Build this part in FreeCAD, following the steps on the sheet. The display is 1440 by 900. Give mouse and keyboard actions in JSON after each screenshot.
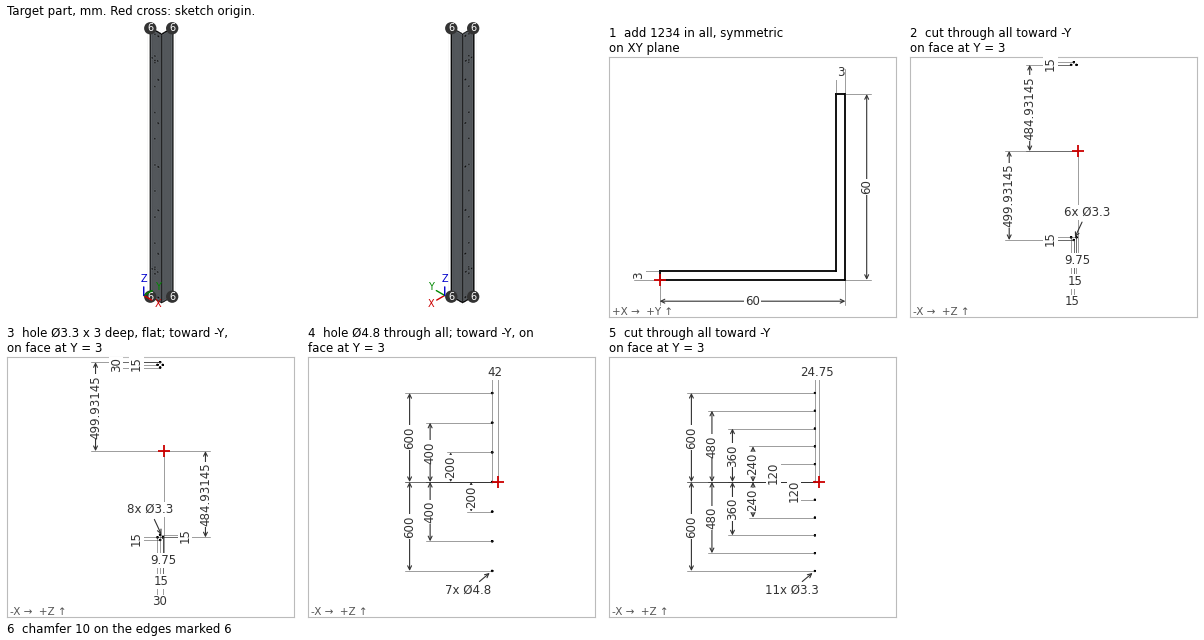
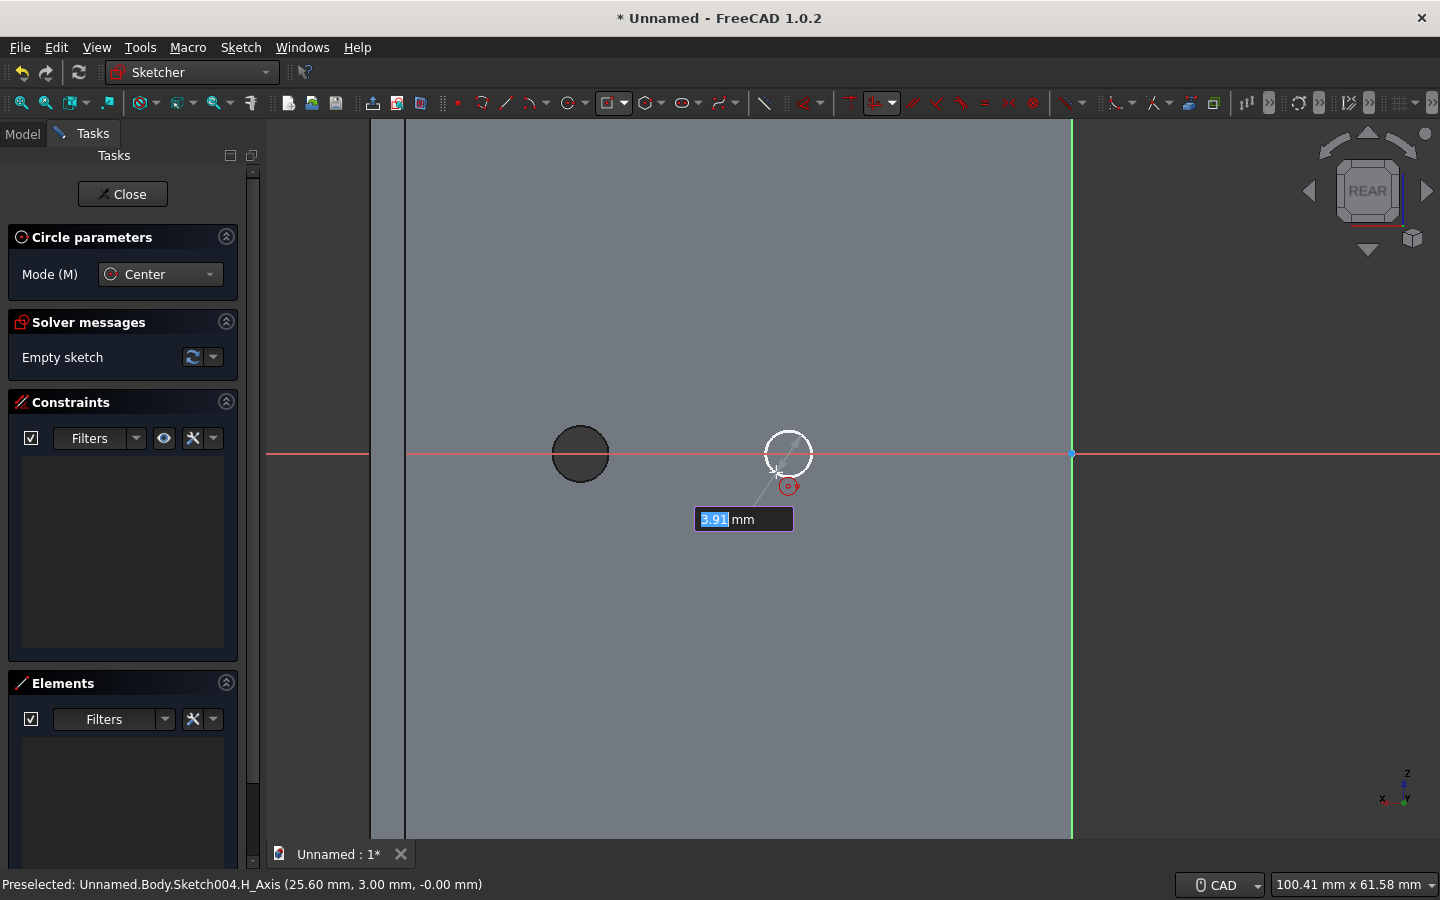
{"action": "type", "text": "3.3"}
{"action": "key", "text": "Return"}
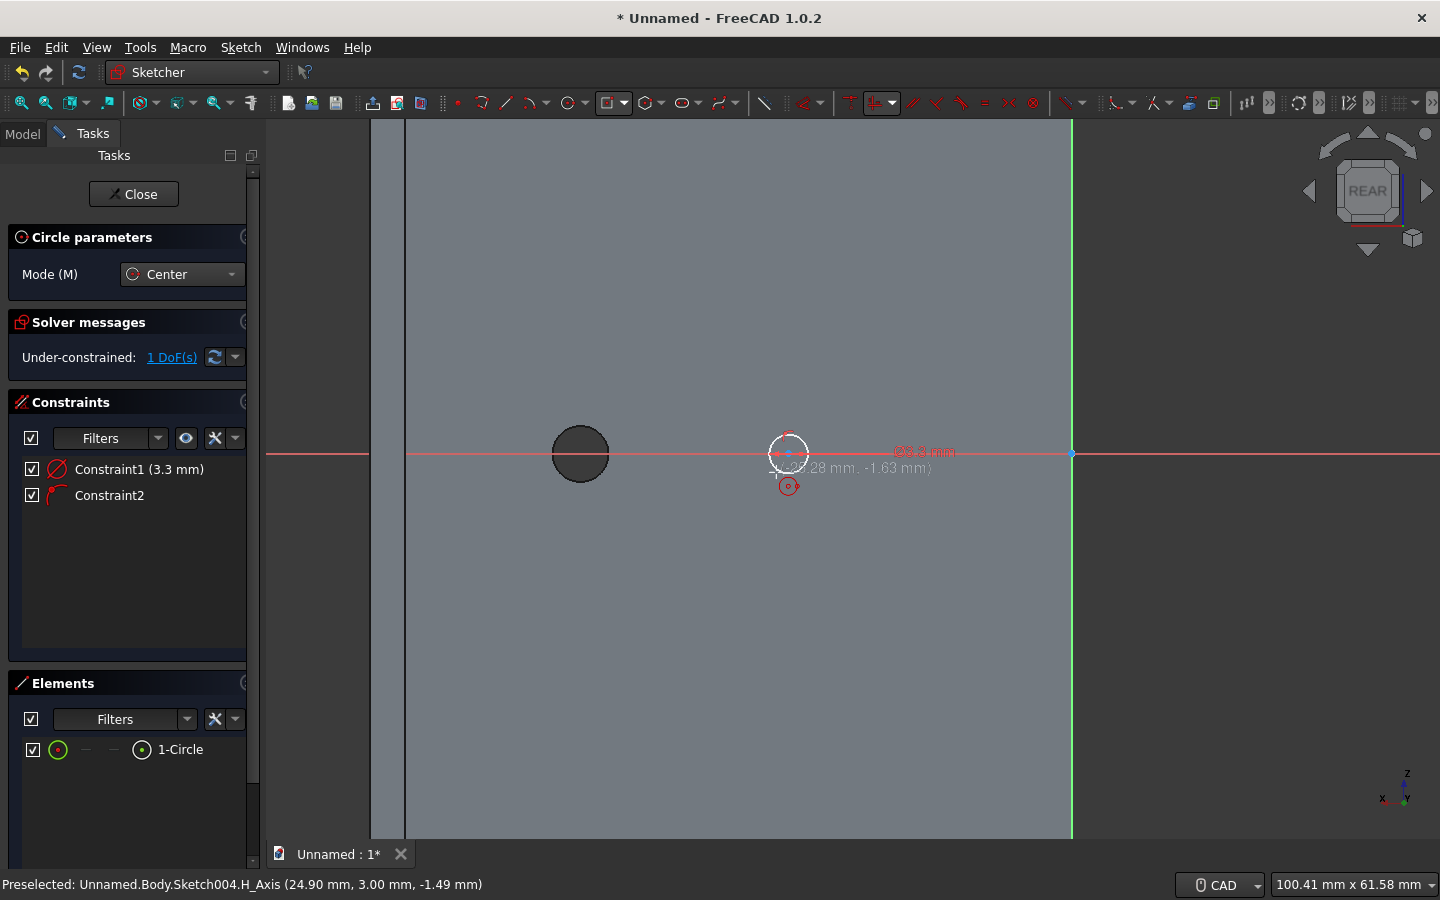
{"action": "scroll", "coordinate": [779, 480], "scroll_direction": "down", "scroll_amount": 16}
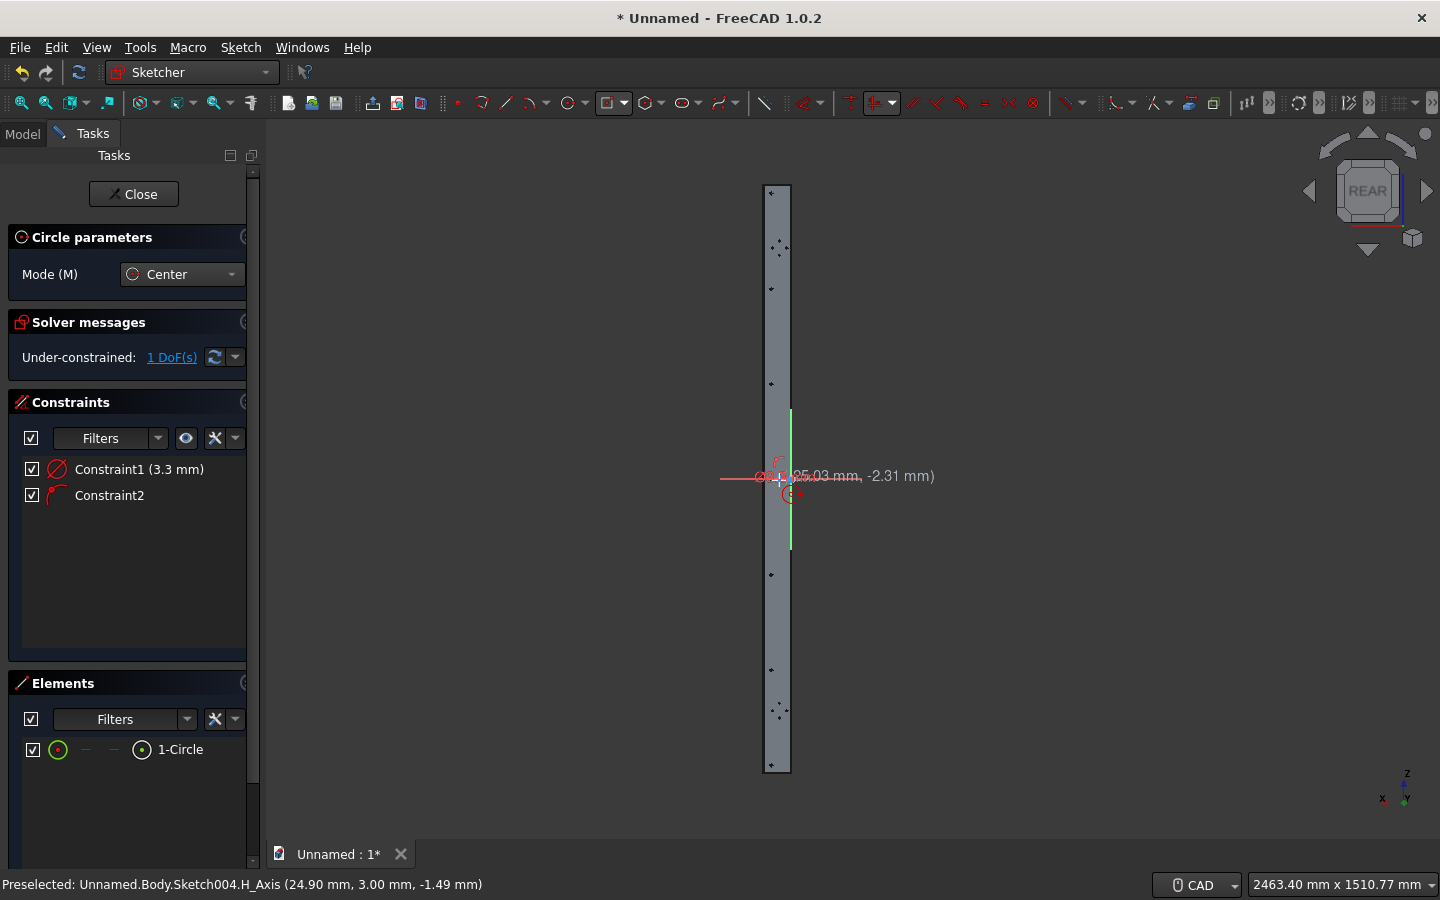
{"action": "scroll", "coordinate": [780, 537], "scroll_direction": "up", "scroll_amount": 17}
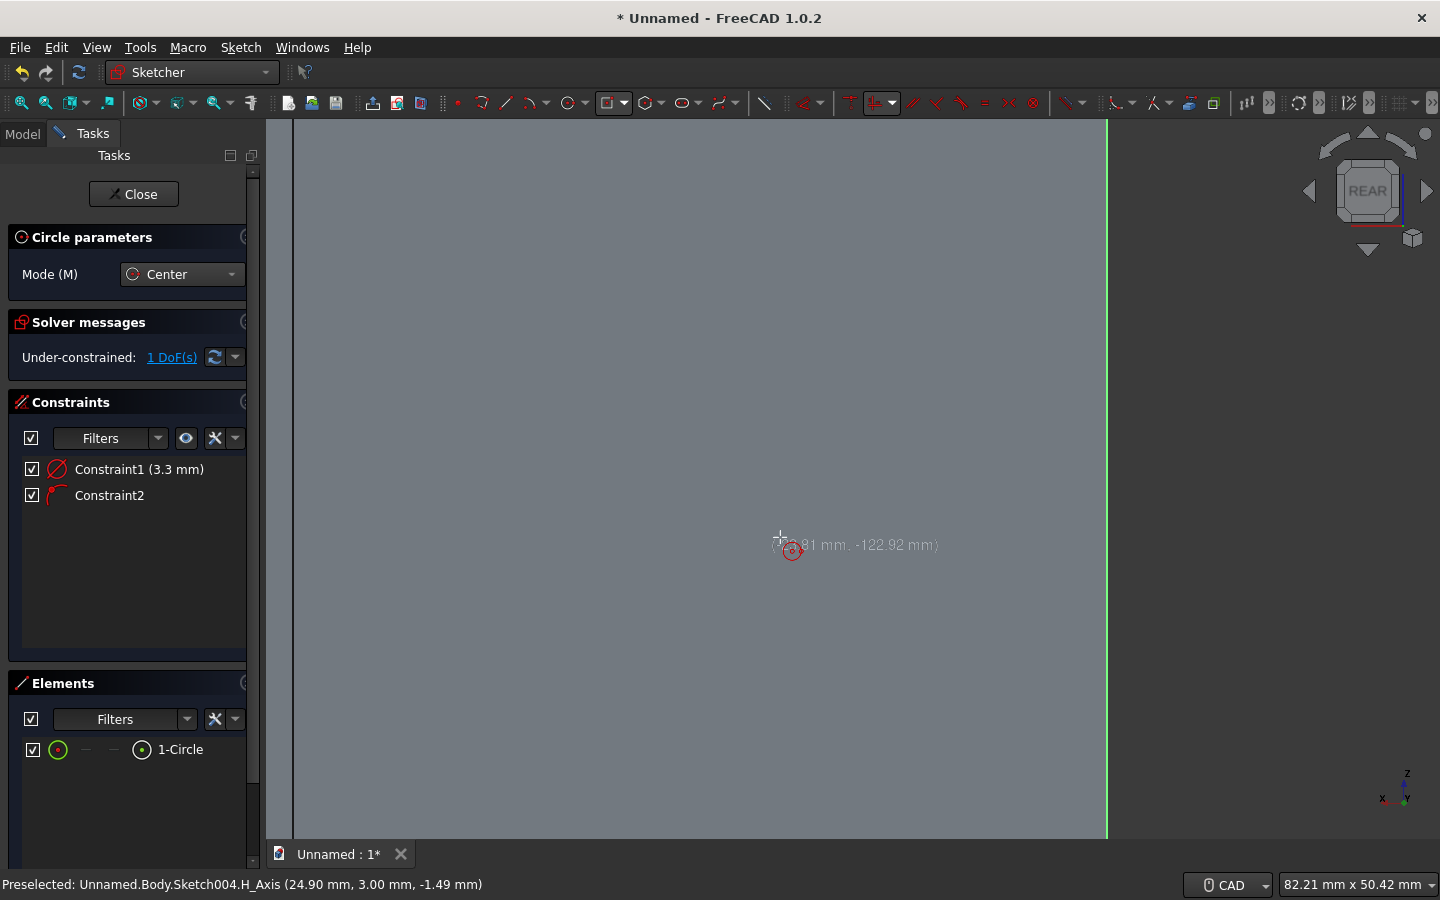
{"action": "scroll", "coordinate": [780, 537], "scroll_direction": "down", "scroll_amount": 17}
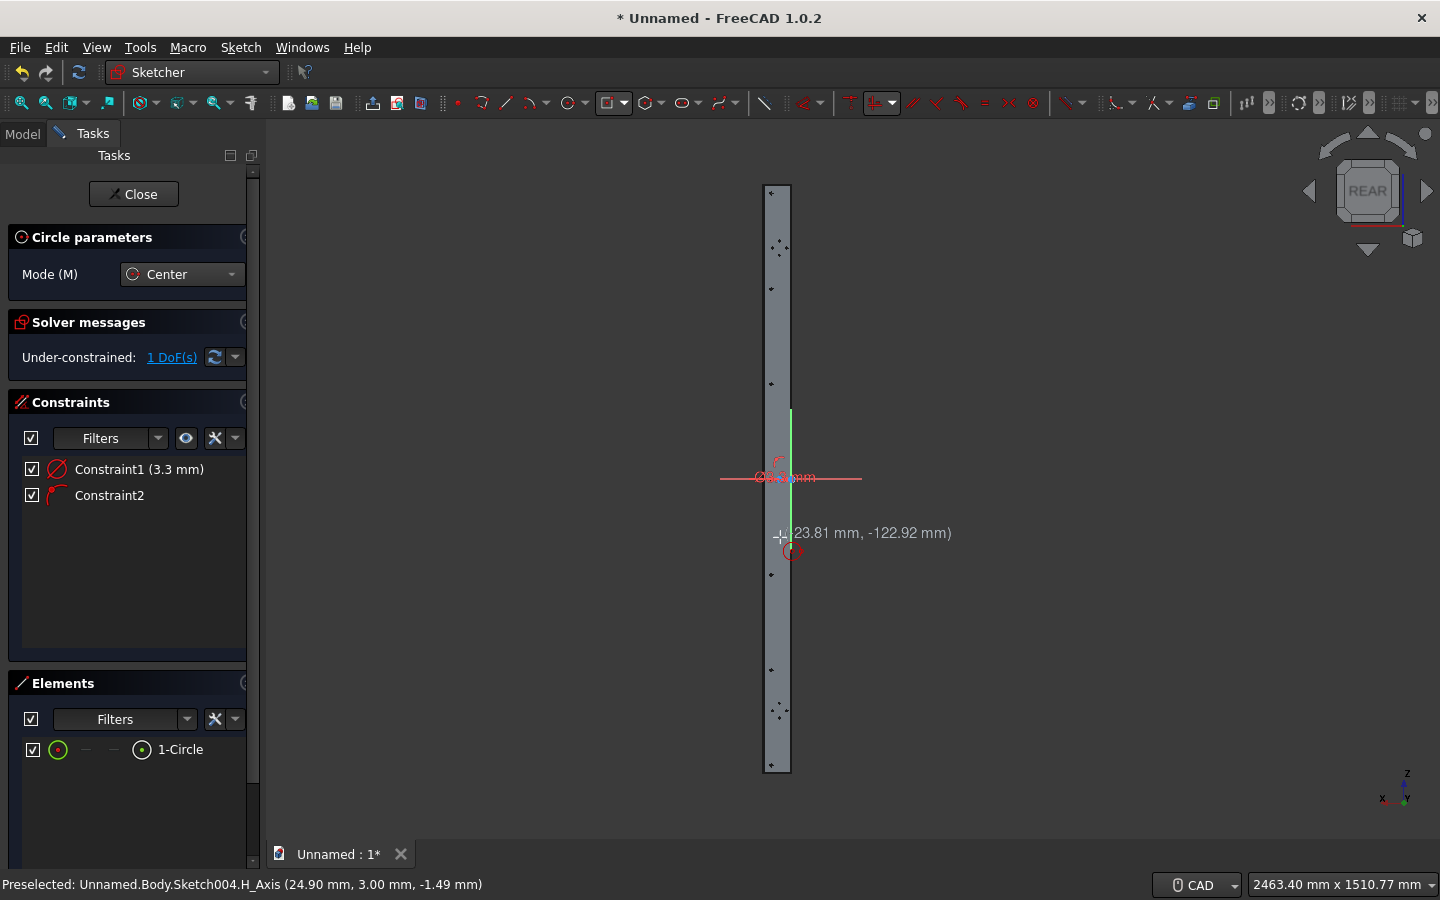
{"action": "scroll", "coordinate": [780, 537], "scroll_direction": "up", "scroll_amount": 2}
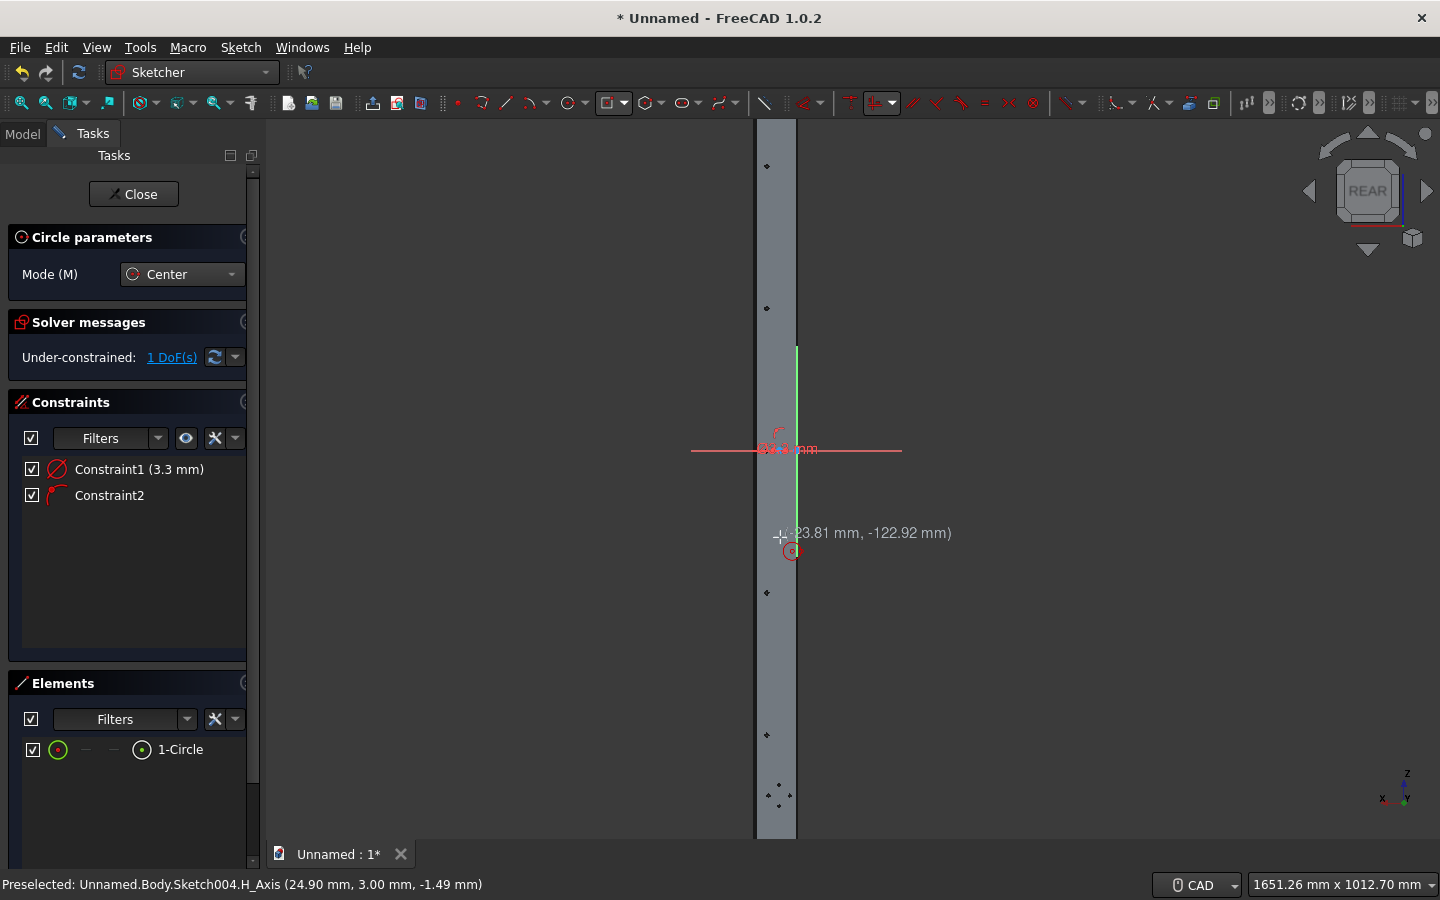
{"action": "left_click", "coordinate": [779, 536]}
{"action": "mouse_move", "coordinate": [780, 535]}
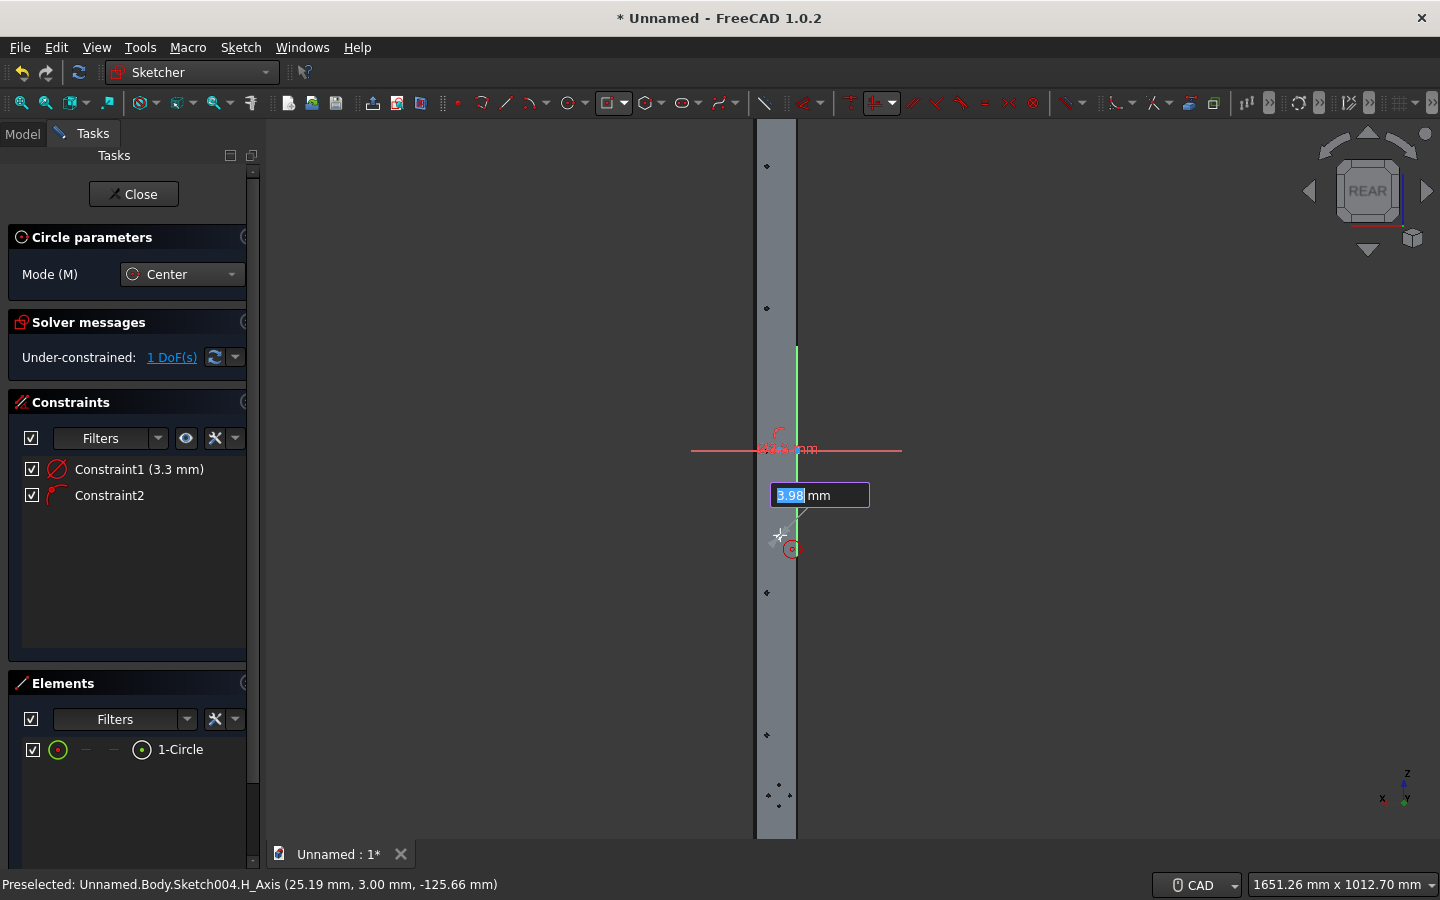
{"action": "type", "text": "3.3"}
{"action": "key", "text": "Return"}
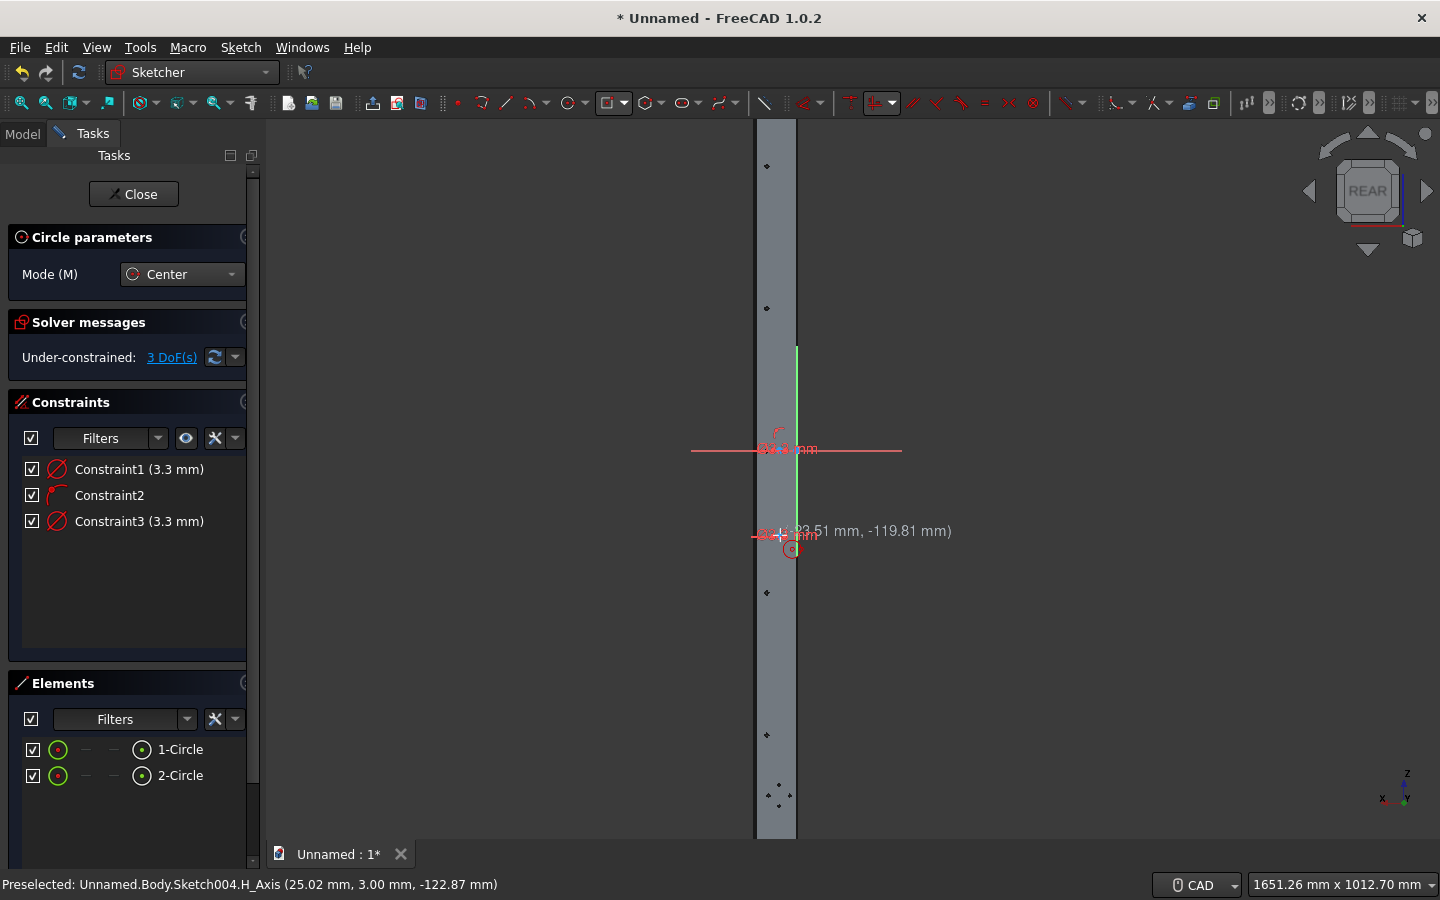
{"action": "scroll", "coordinate": [779, 621], "scroll_direction": "up", "scroll_amount": 15}